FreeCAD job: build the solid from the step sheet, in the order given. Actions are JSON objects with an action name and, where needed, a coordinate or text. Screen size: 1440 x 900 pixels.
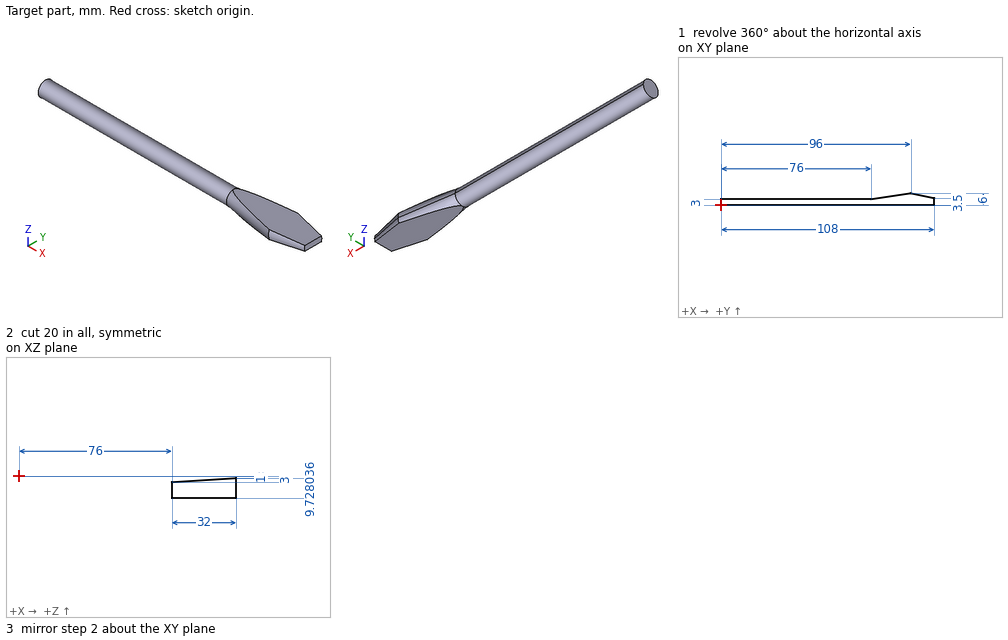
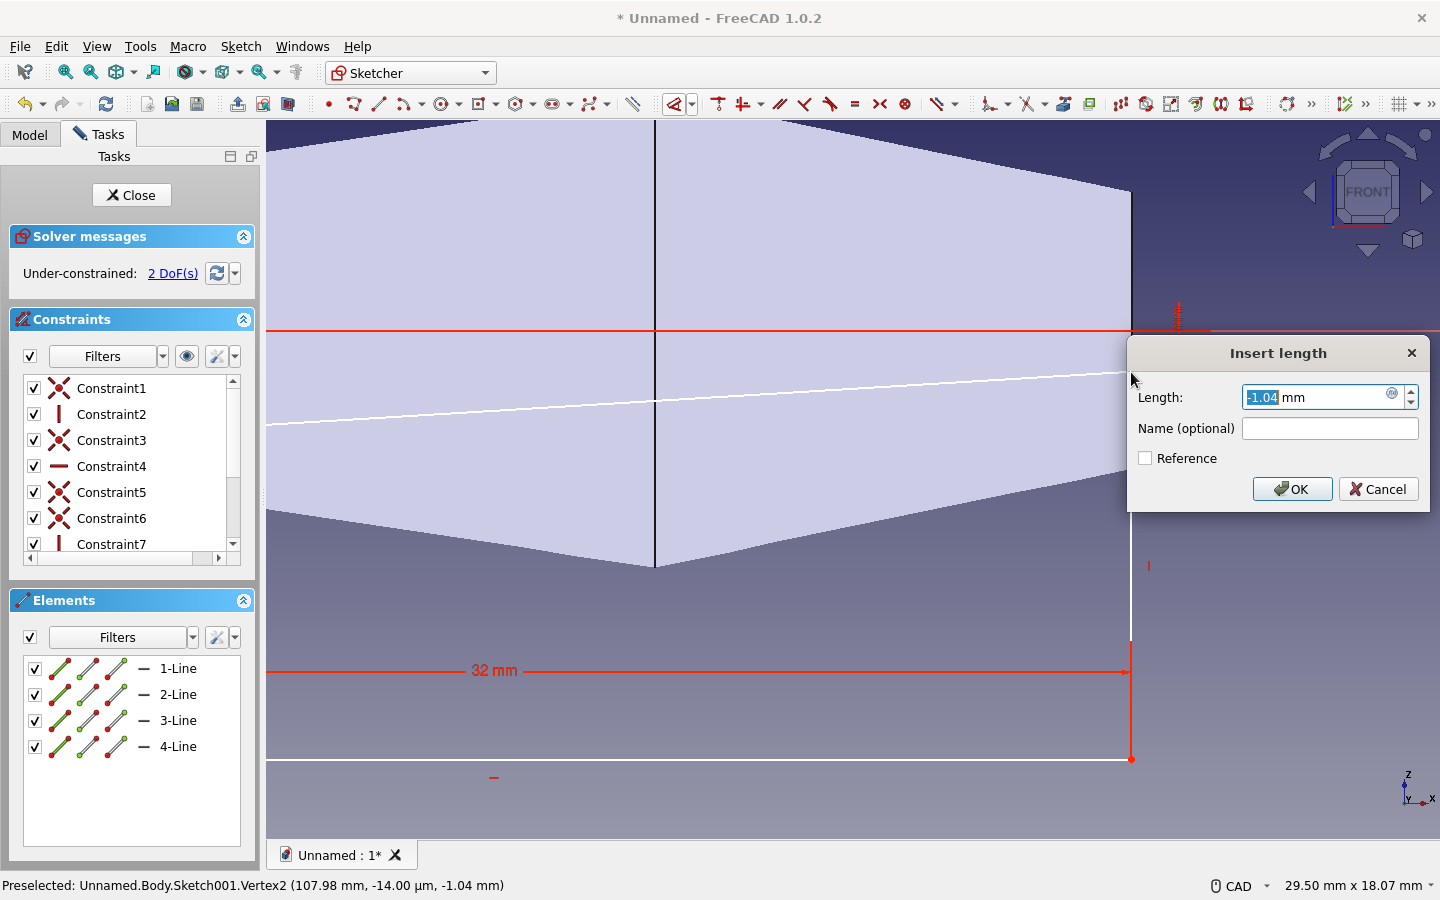
{"action": "type", "text": "-1"}
{"action": "key", "text": "Return"}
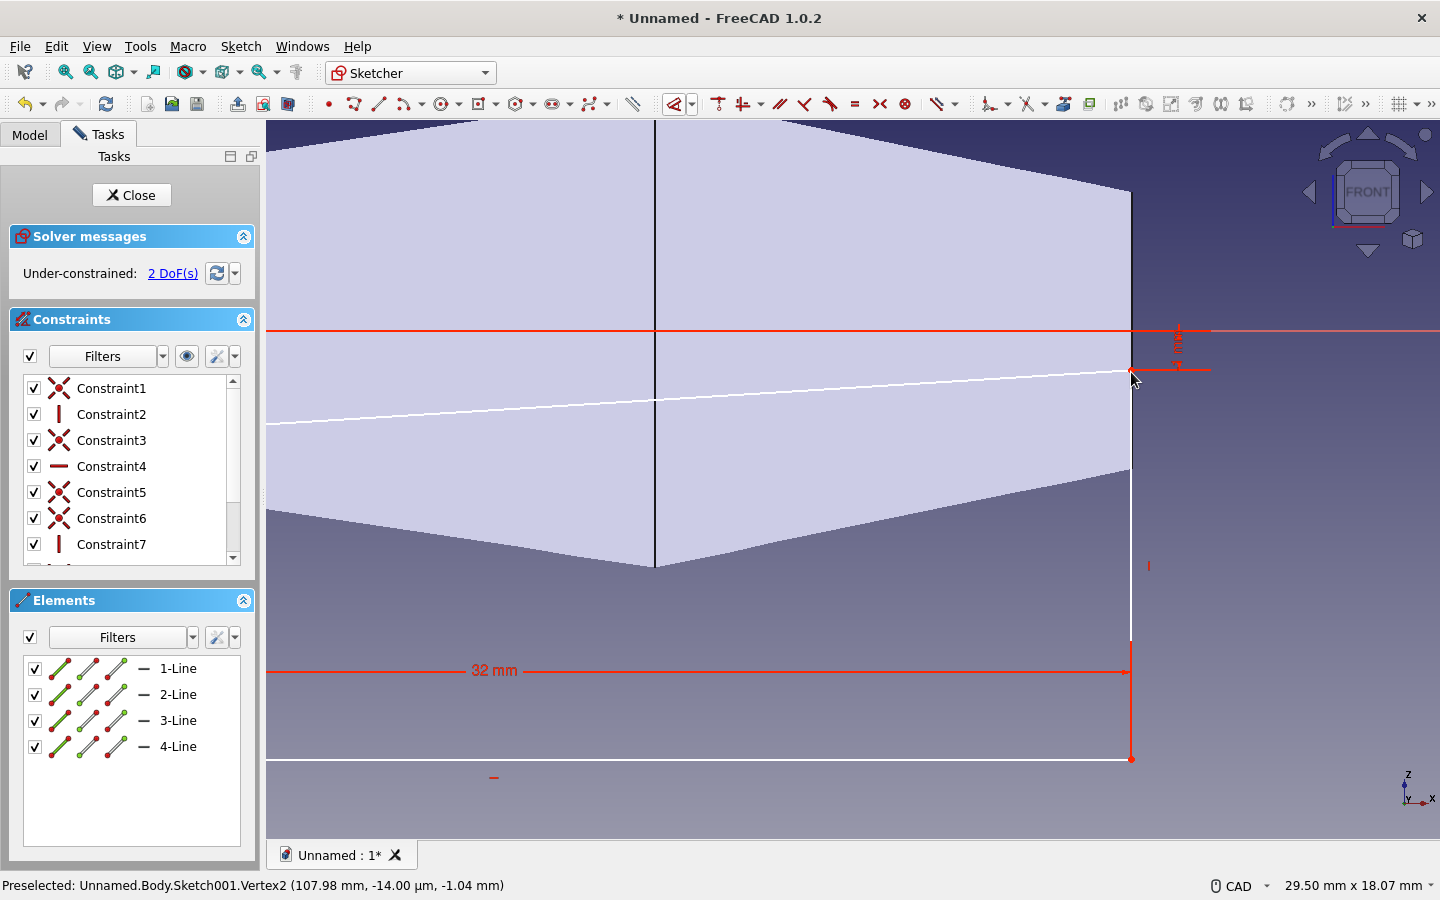
{"action": "scroll", "coordinate": [1136, 377], "scroll_direction": "down", "scroll_amount": 3}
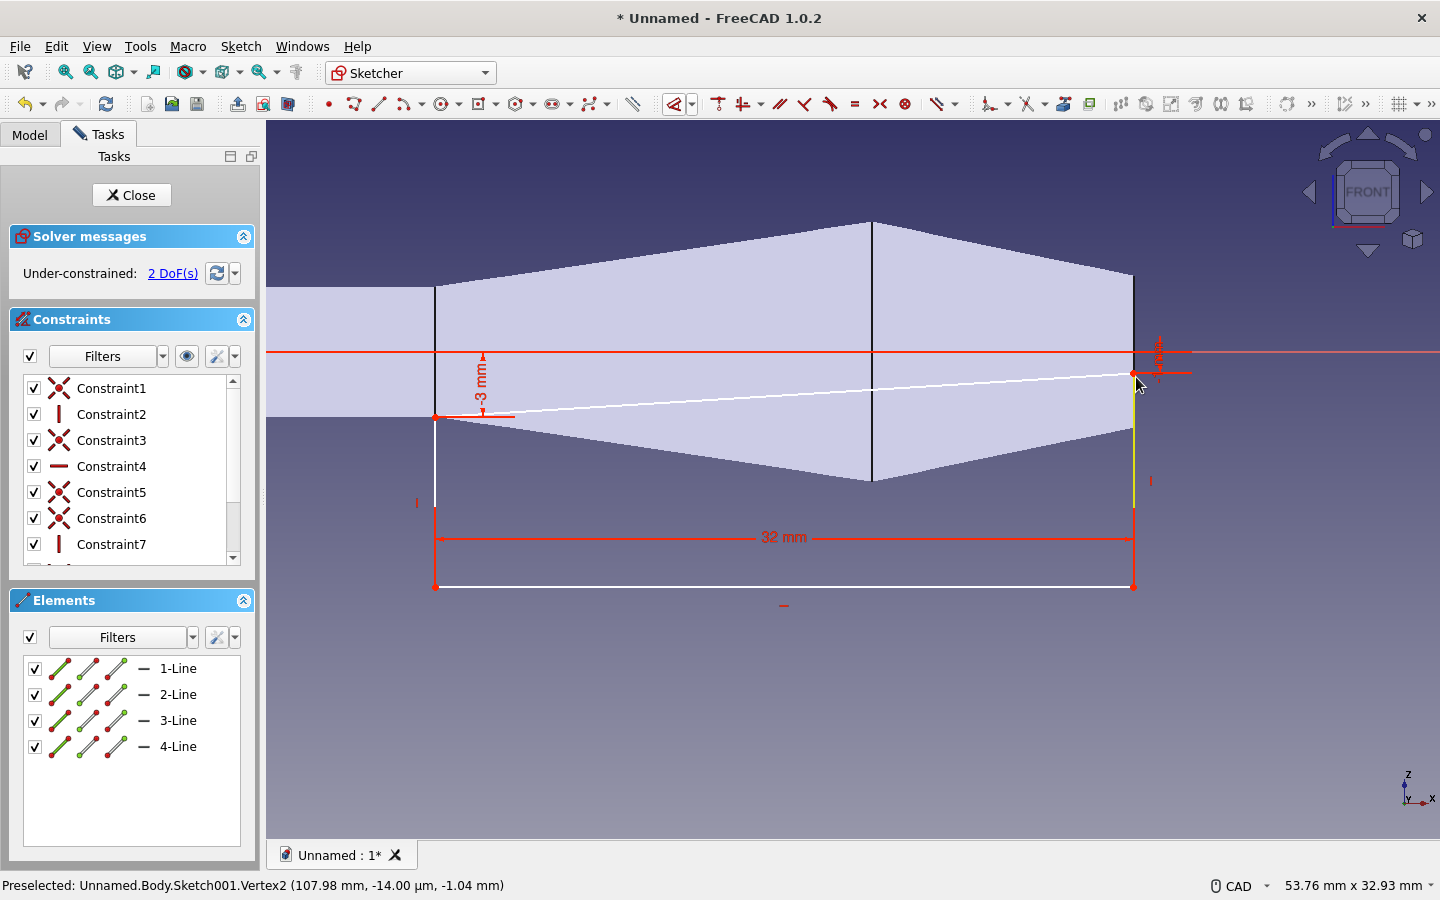
{"action": "left_click", "coordinate": [435, 417]}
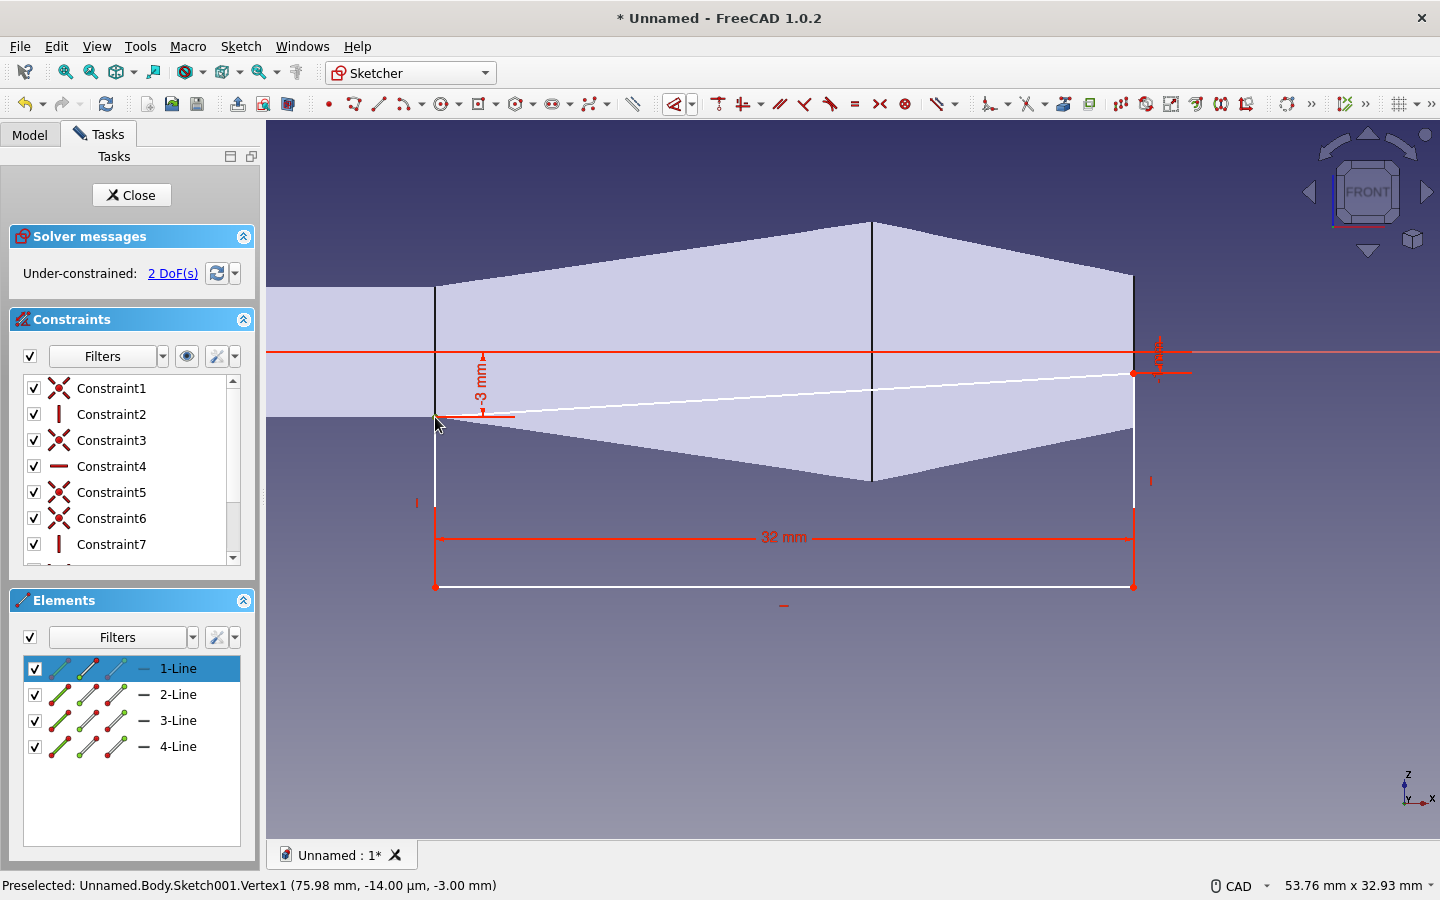
{"action": "key", "text": "l"}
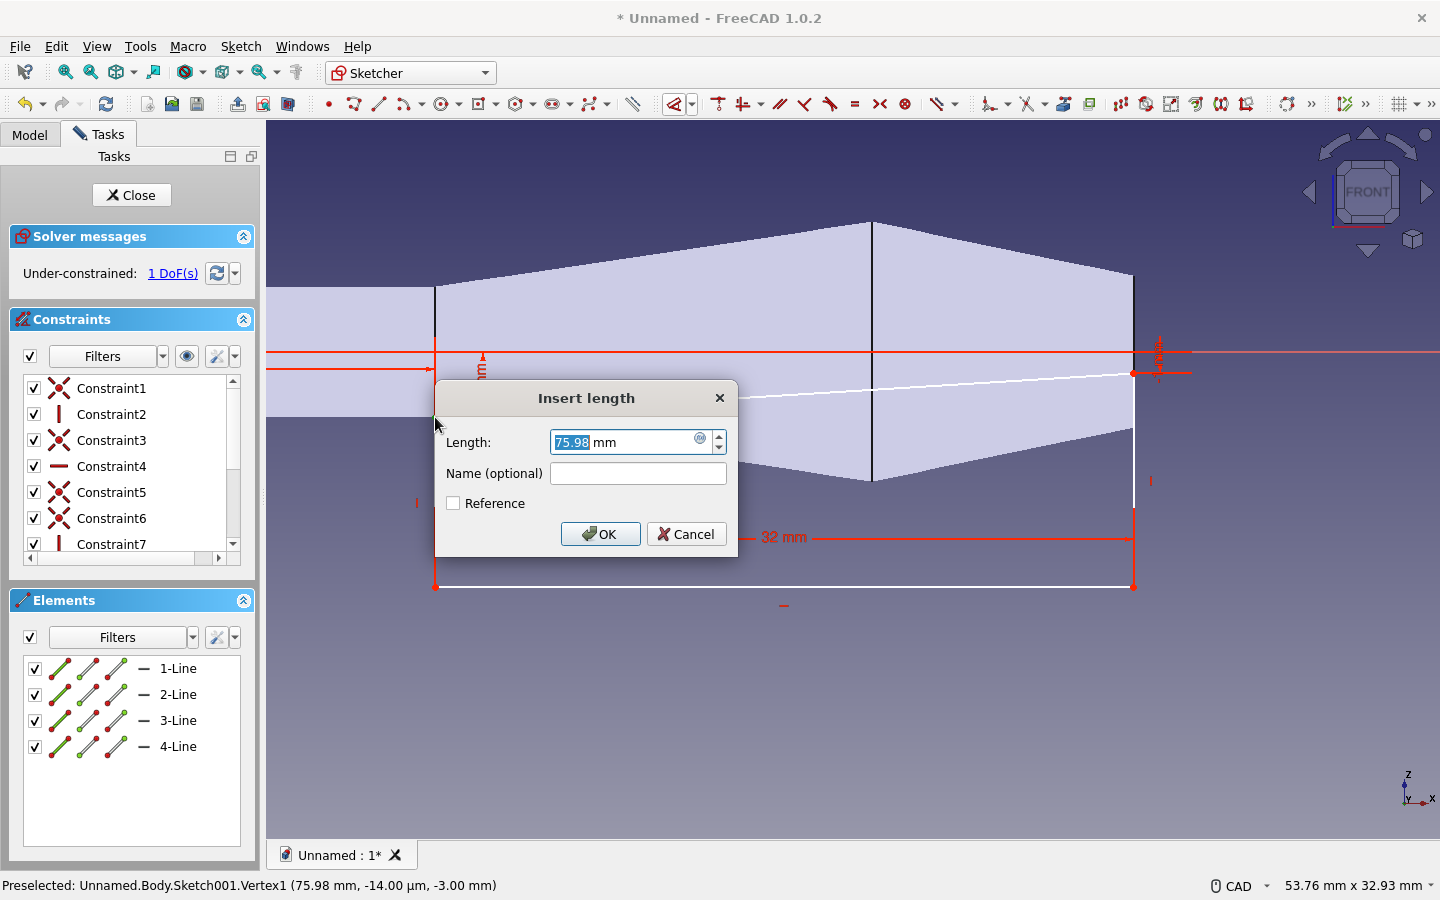
{"action": "type", "text": "76"}
{"action": "key", "text": "Return"}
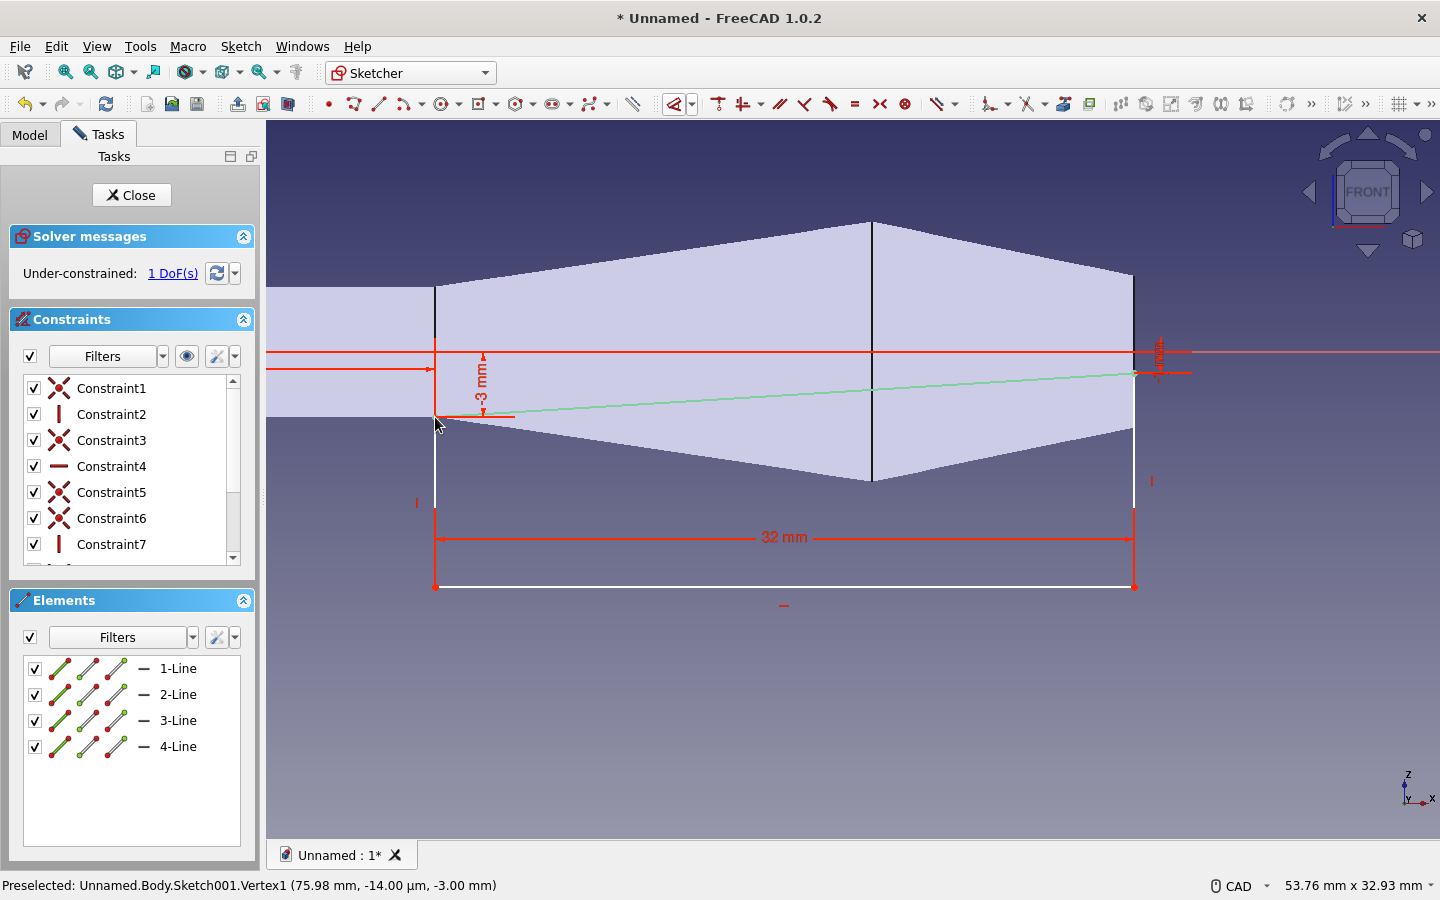
{"action": "left_click", "coordinate": [1134, 438]}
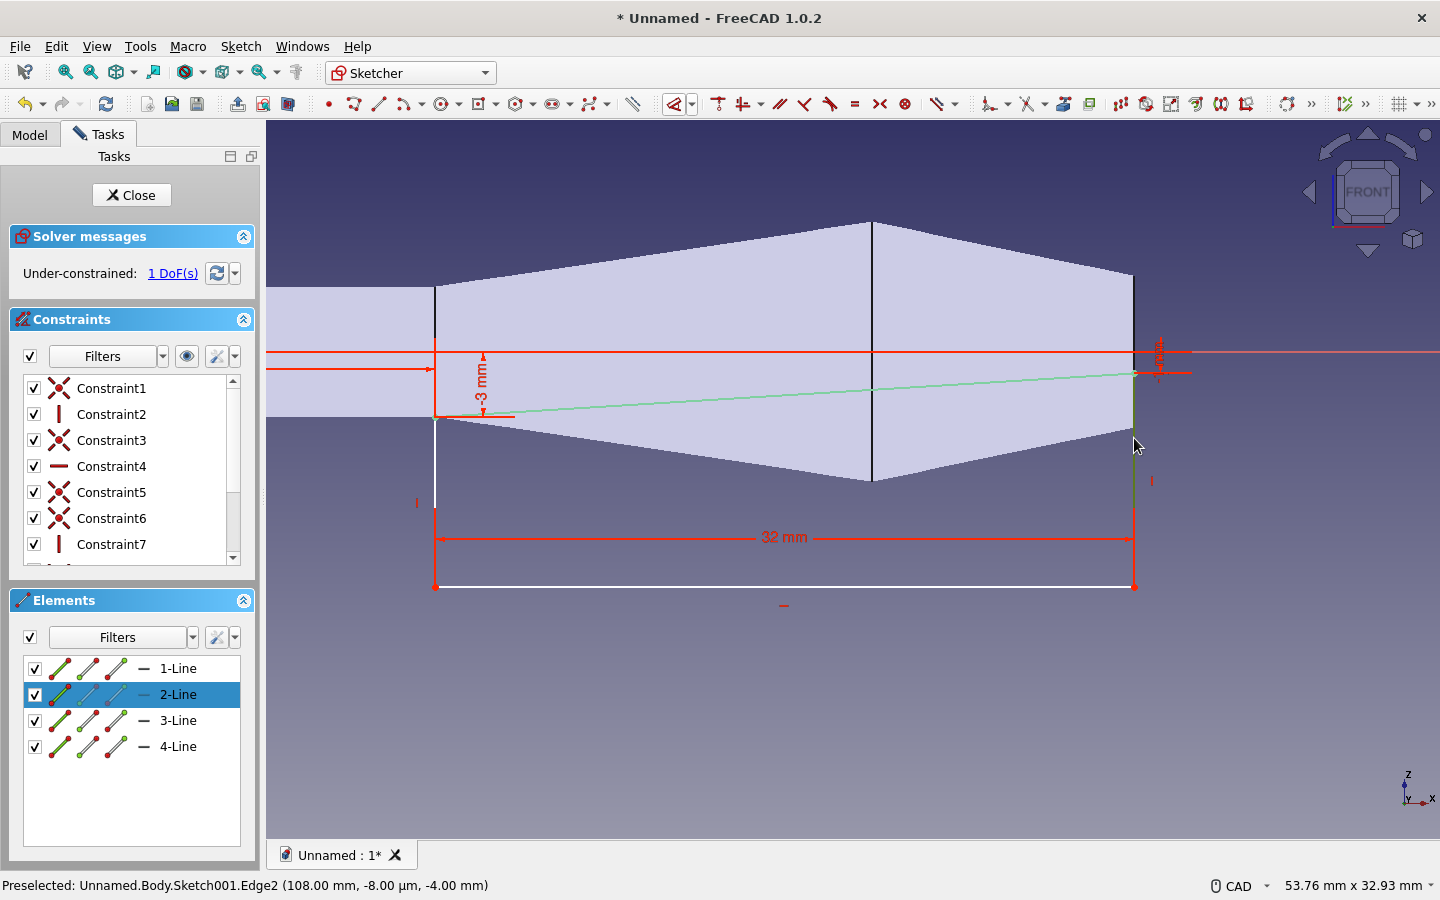
{"action": "key", "text": "i"}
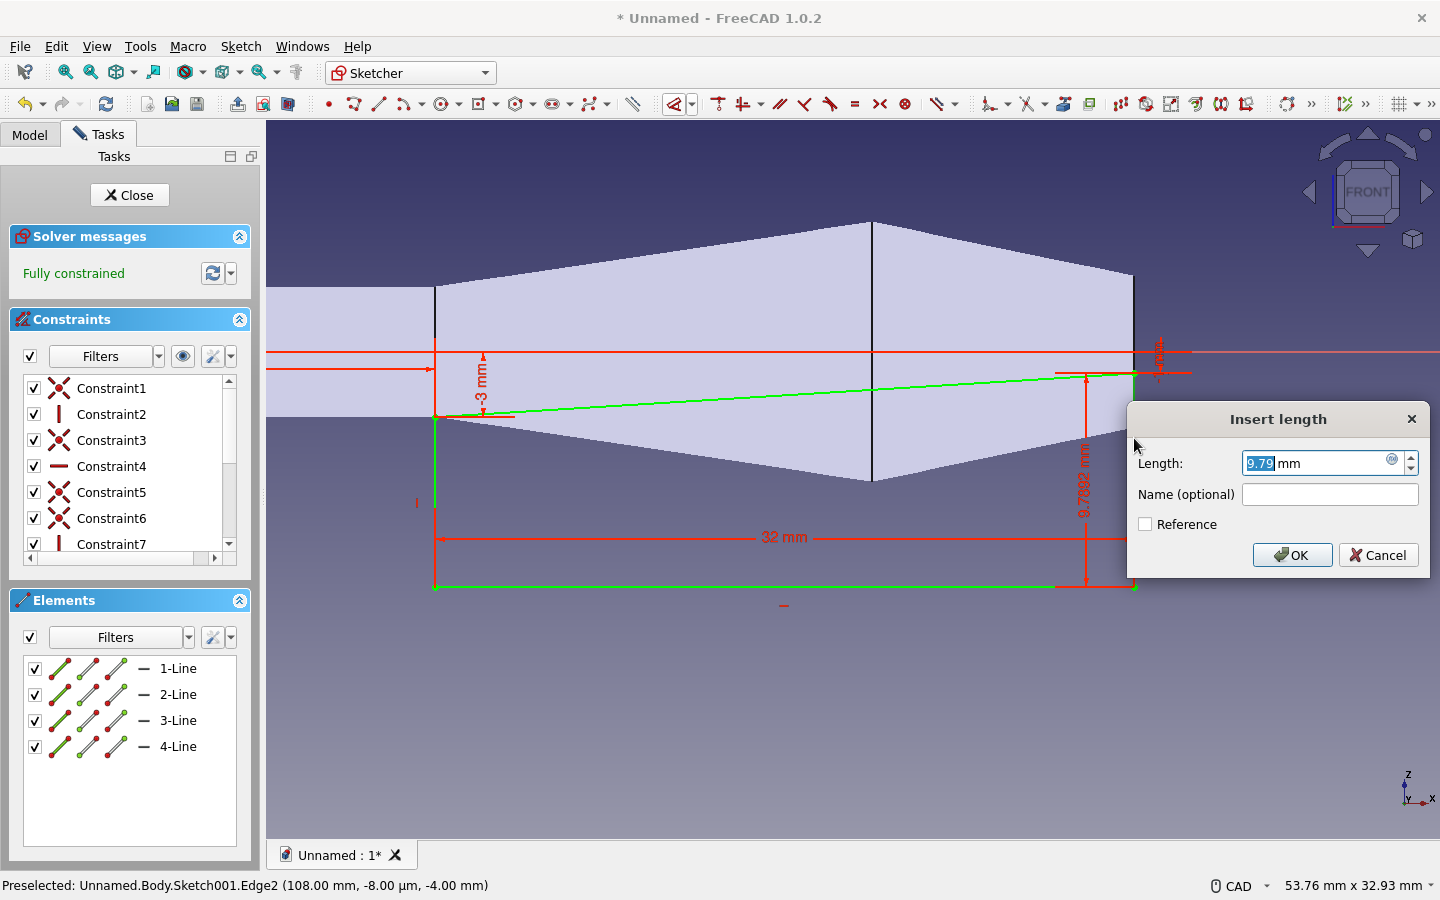
{"action": "type", "text": "9.728036"}
{"action": "key", "text": "Return"}